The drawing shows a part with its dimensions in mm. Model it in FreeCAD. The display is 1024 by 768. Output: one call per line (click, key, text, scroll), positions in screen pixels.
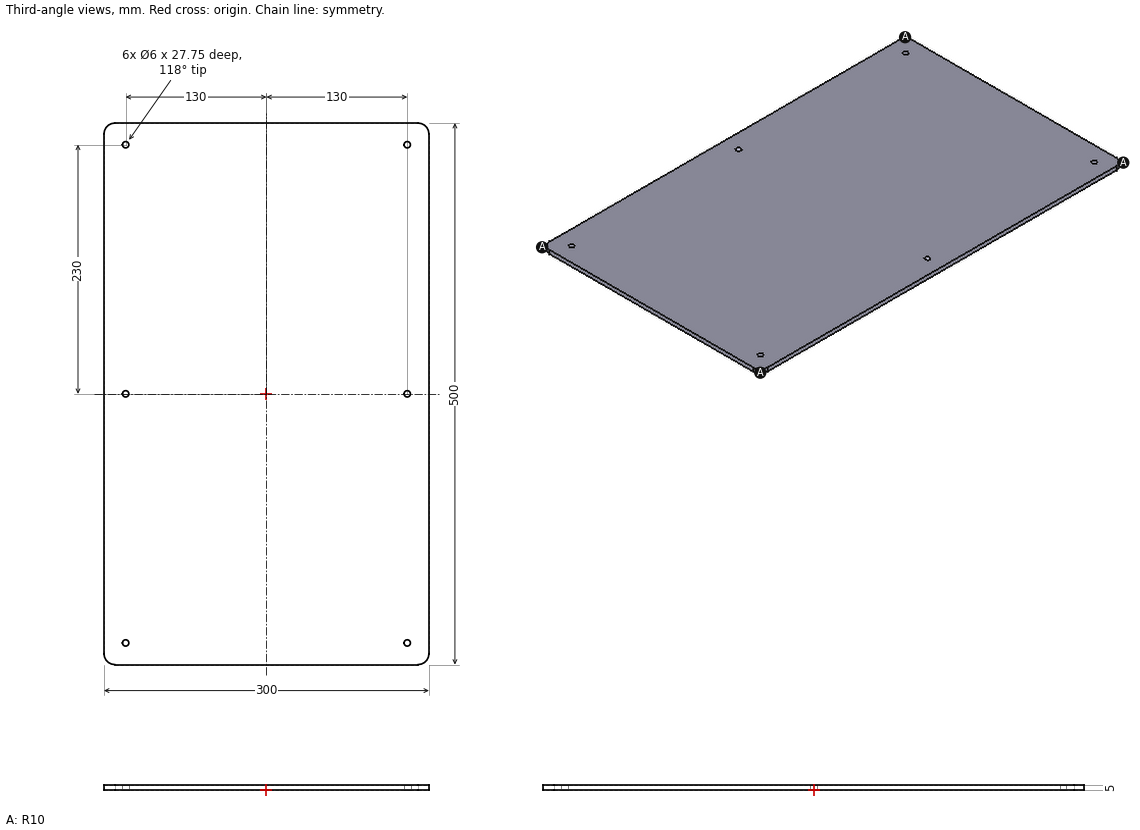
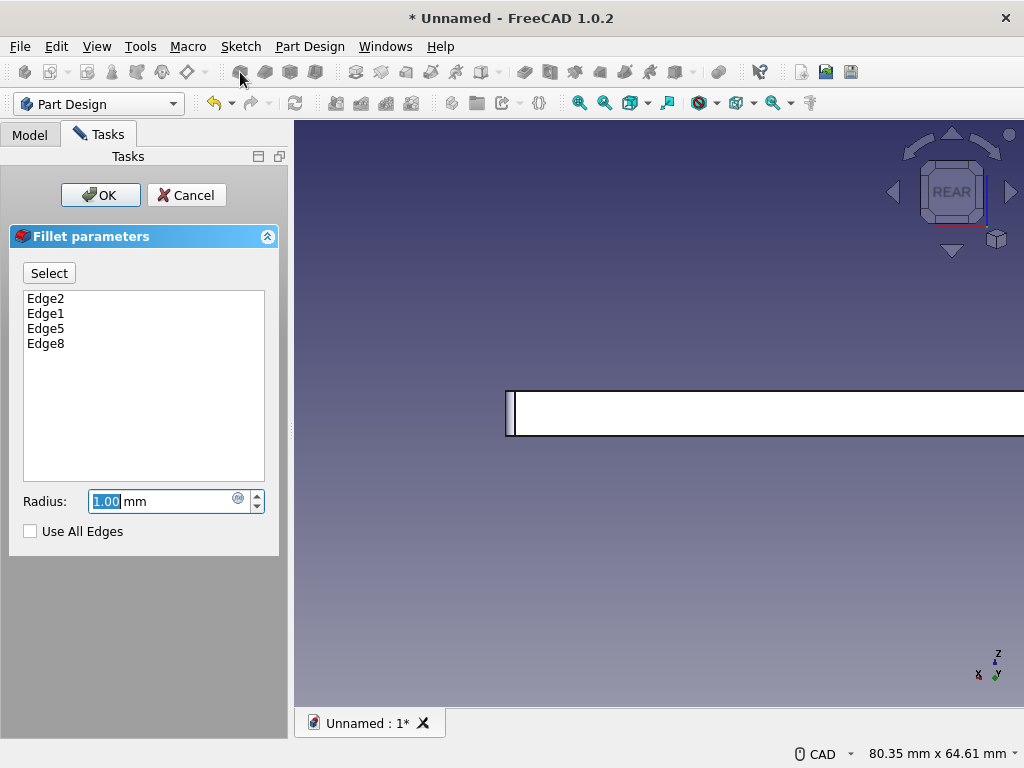
text(10)
key(Tab)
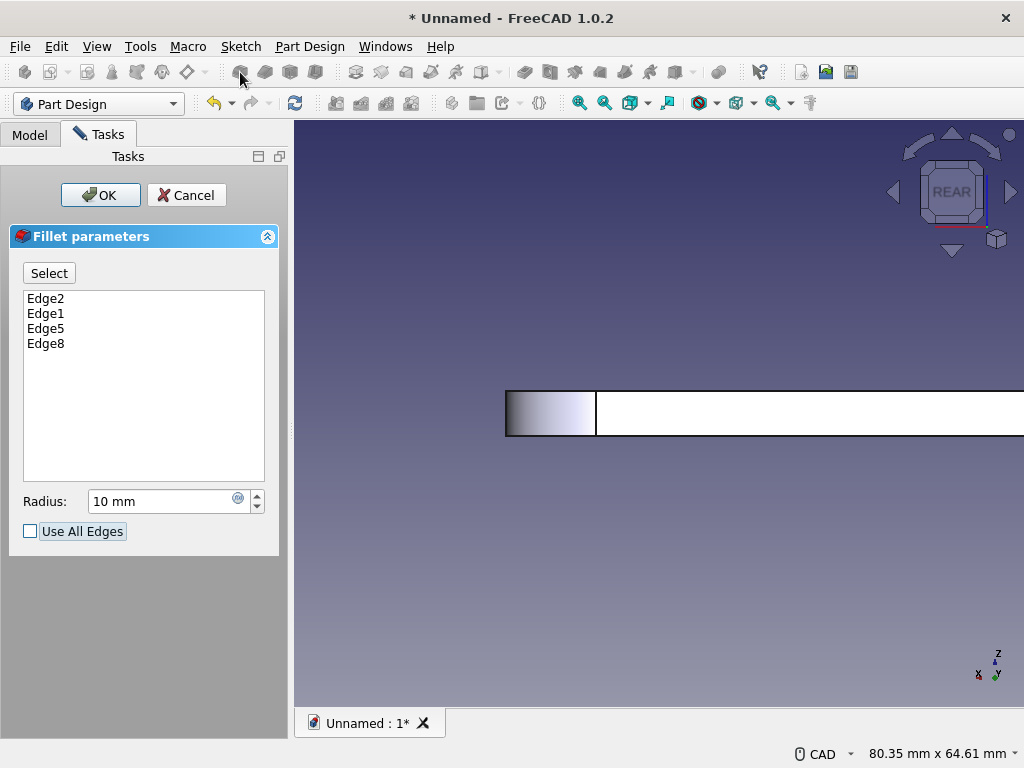
click(101, 195)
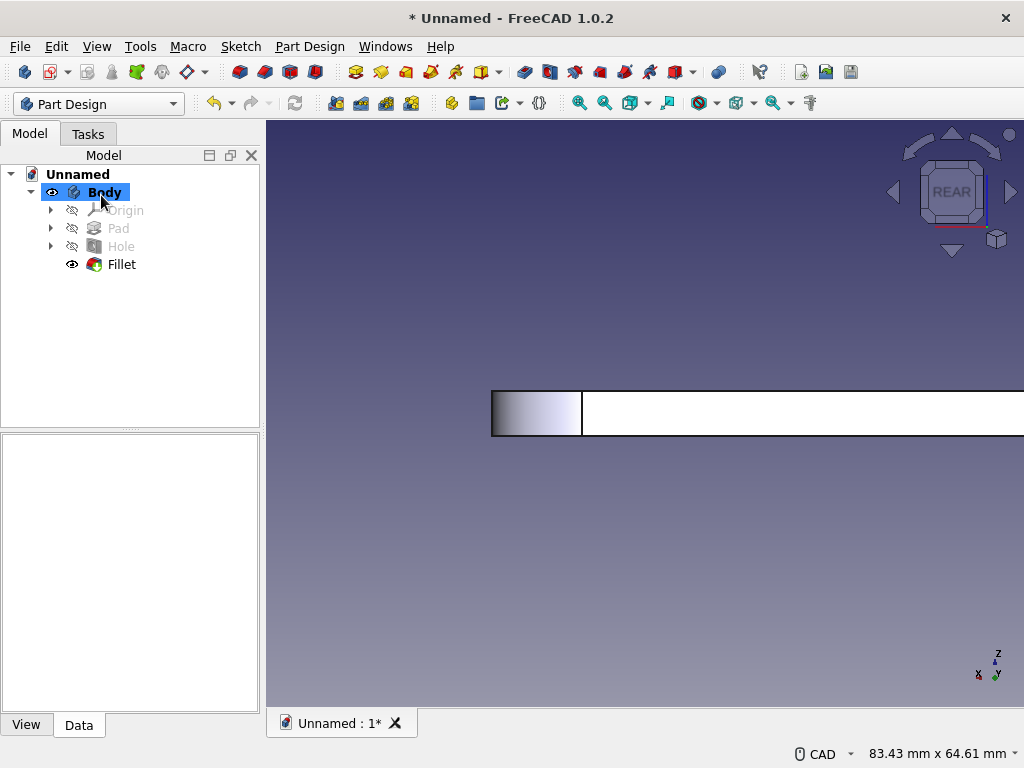
key(0)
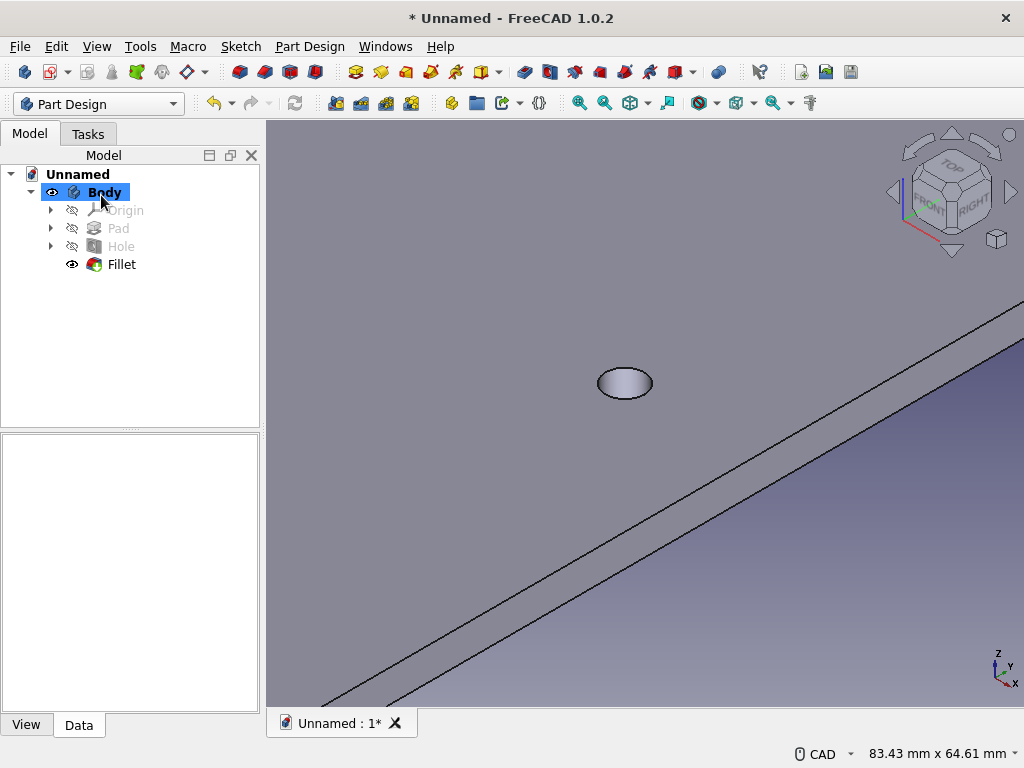
click(580, 104)